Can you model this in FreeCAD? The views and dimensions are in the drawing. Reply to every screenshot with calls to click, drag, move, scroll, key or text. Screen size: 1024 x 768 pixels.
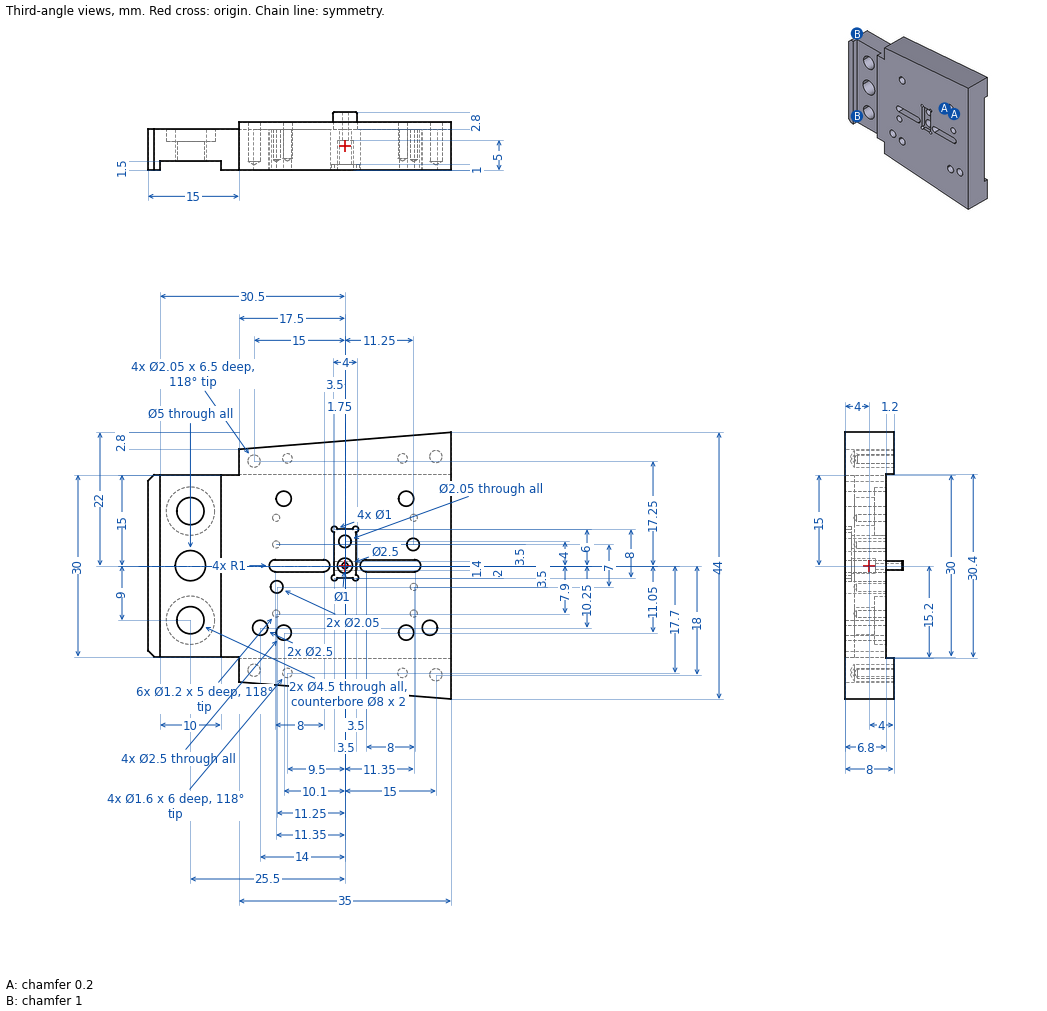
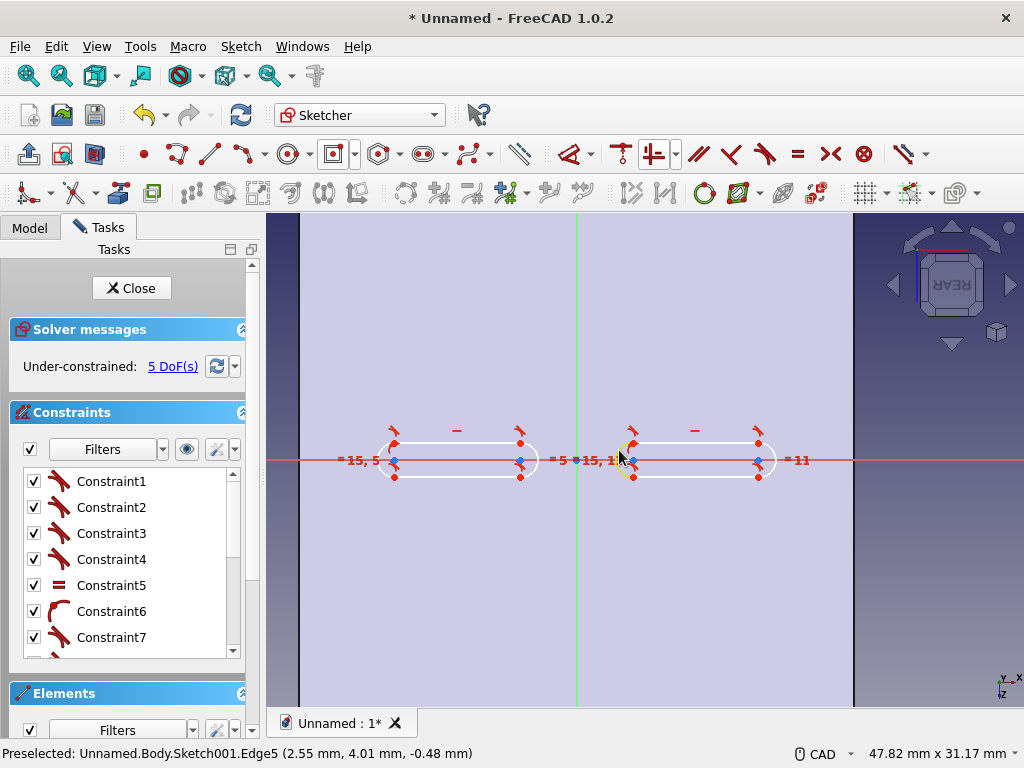
scroll(381, 450, up, 5)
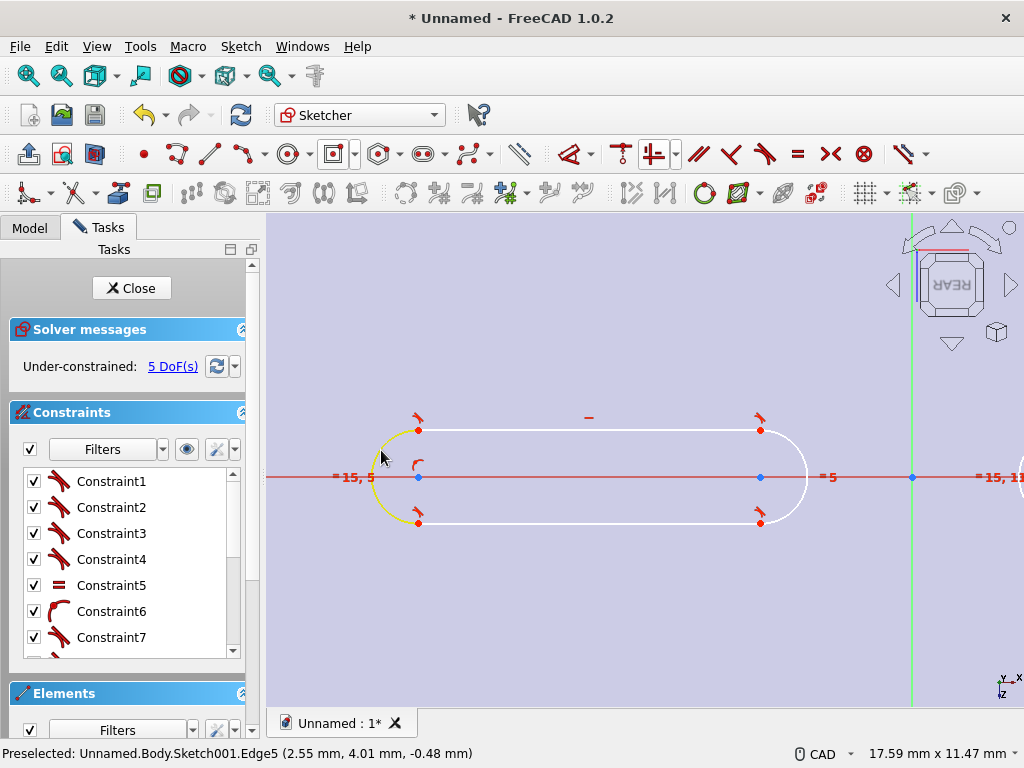
click(381, 450)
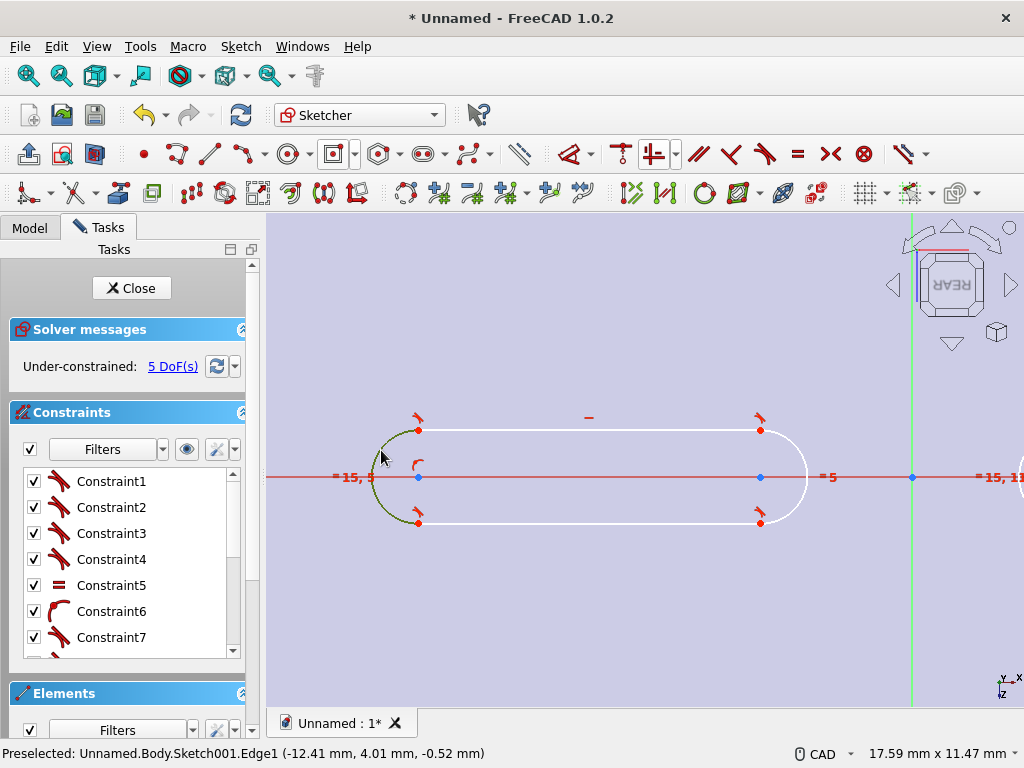
key(k)
key(r)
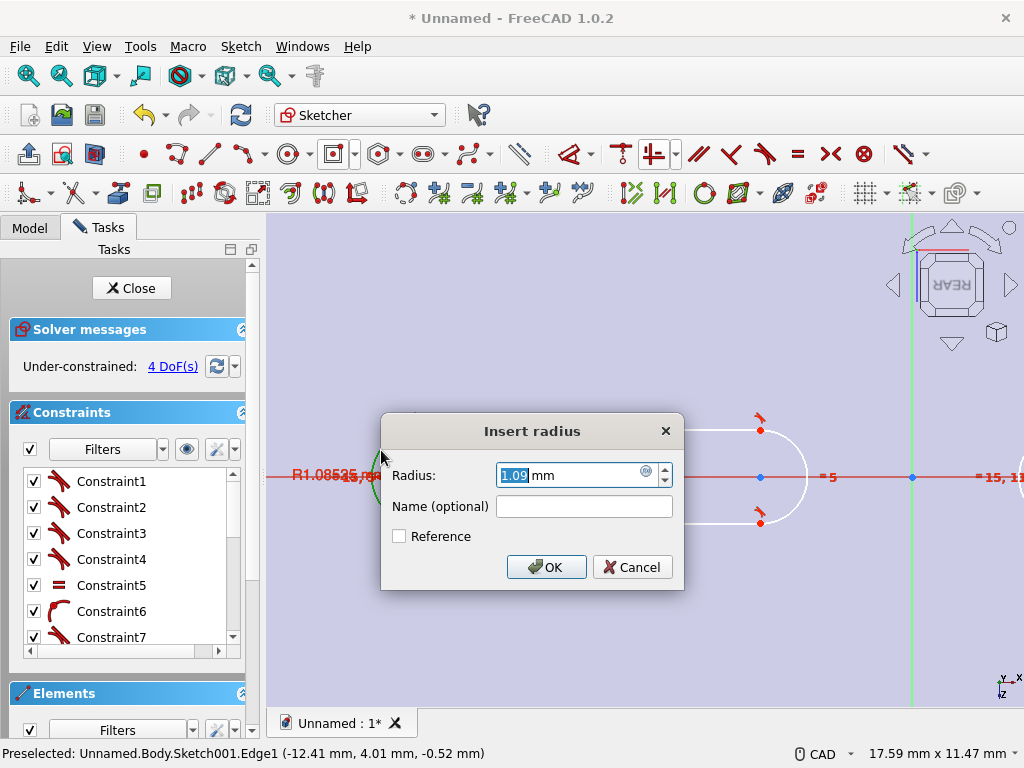
text(1)
key(Return)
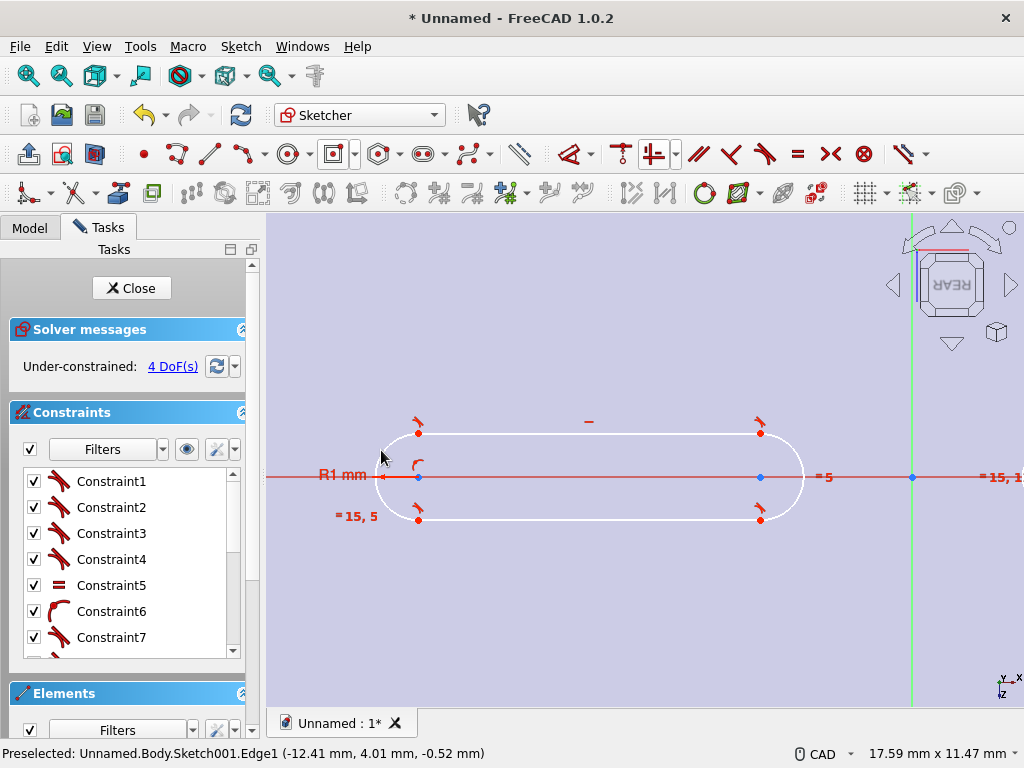
click(521, 434)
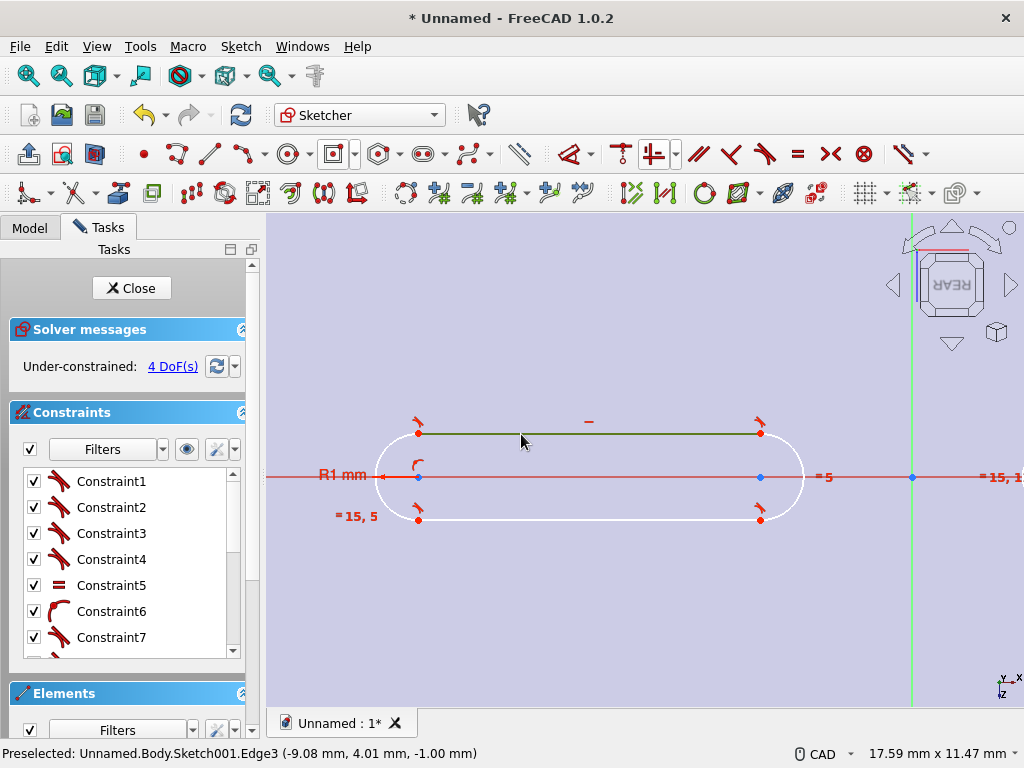
key(l)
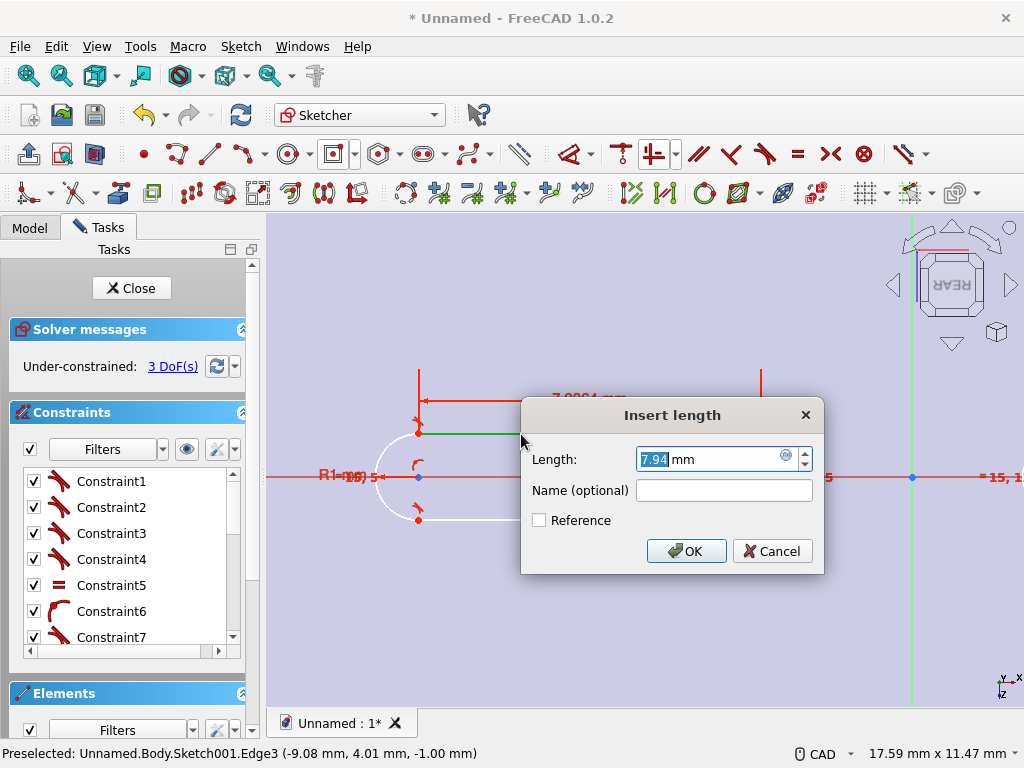
text(8)
key(Return)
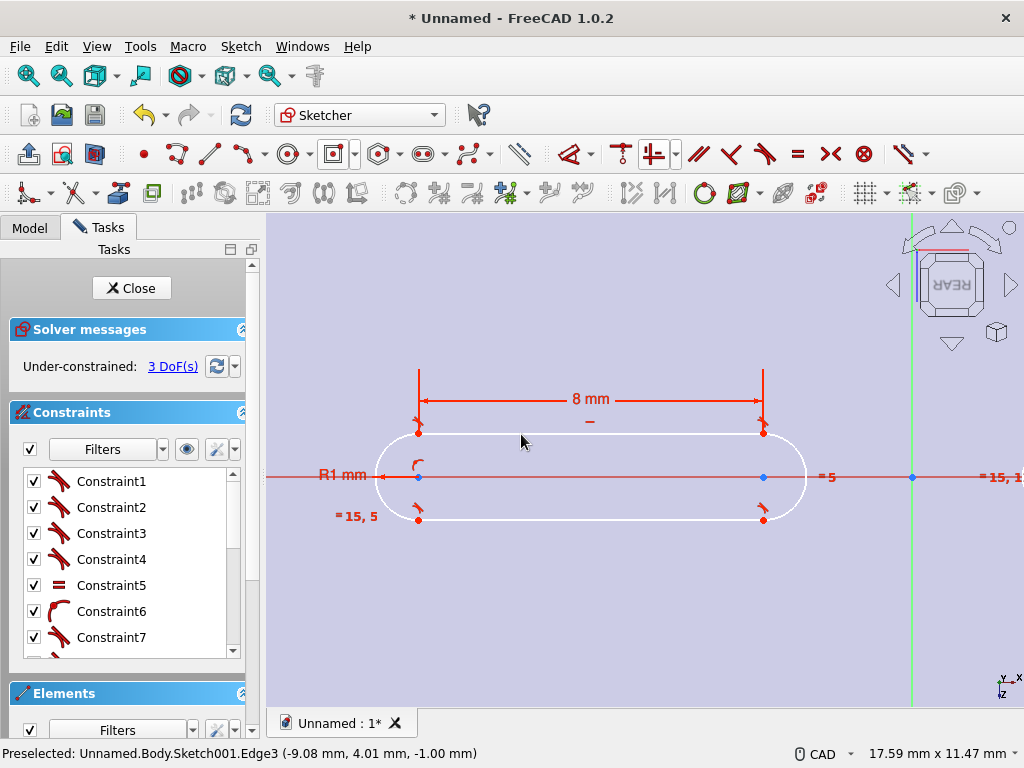
scroll(381, 450, down, 5)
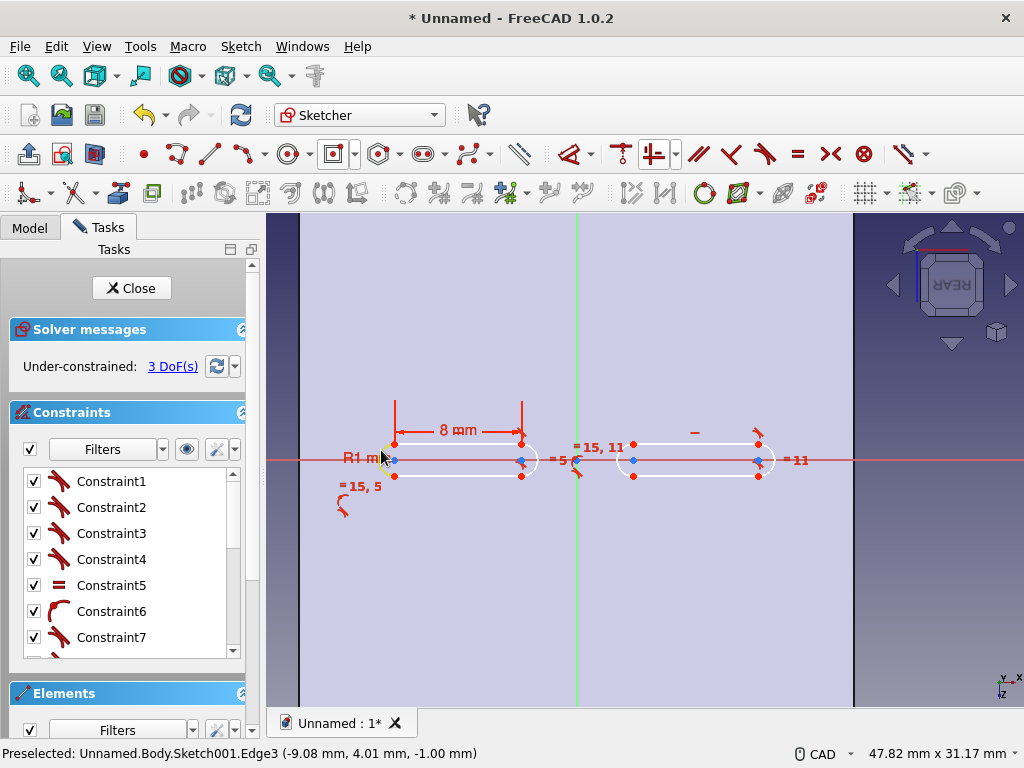
click(671, 444)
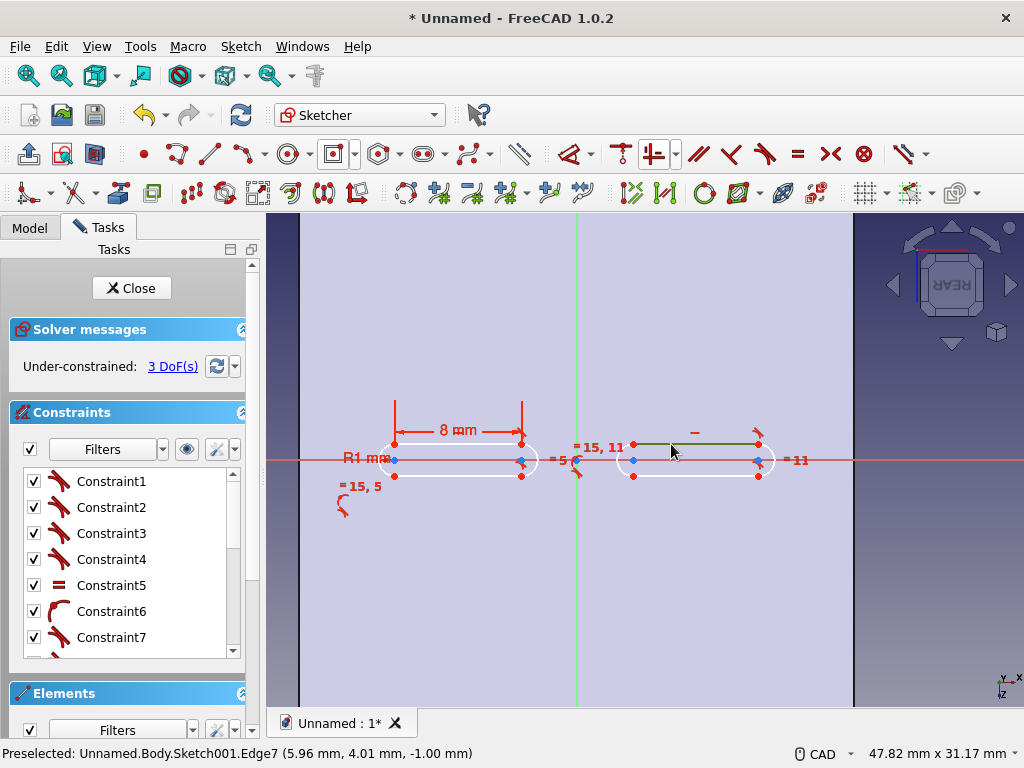
key(l)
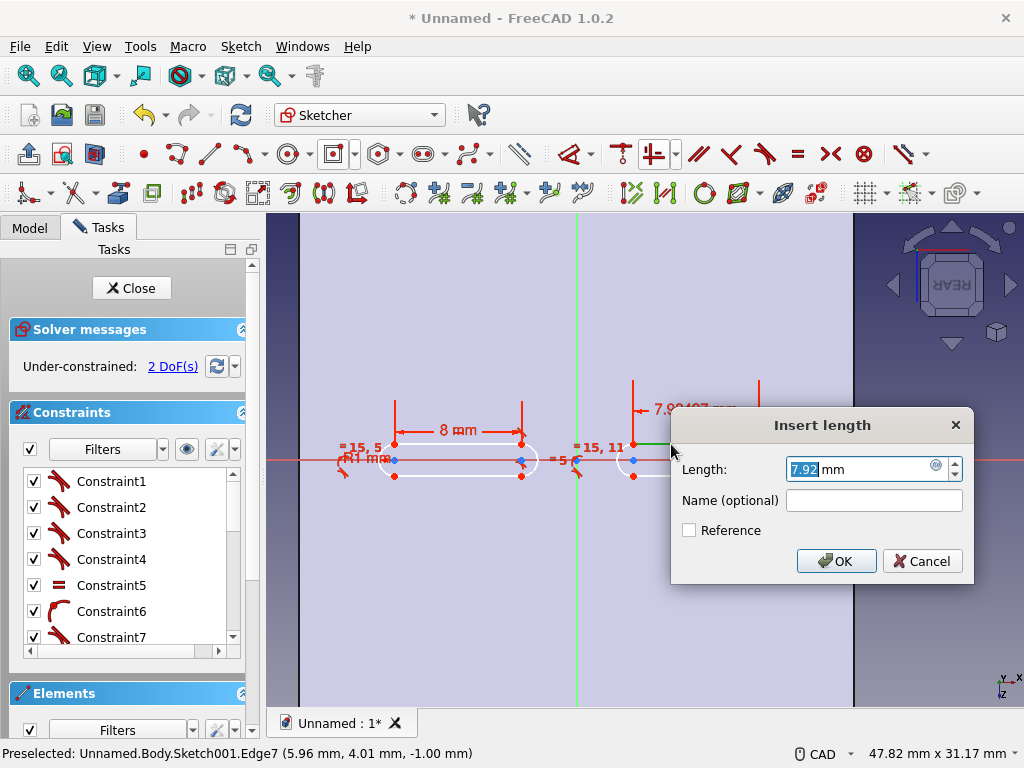
text(8)
key(Return)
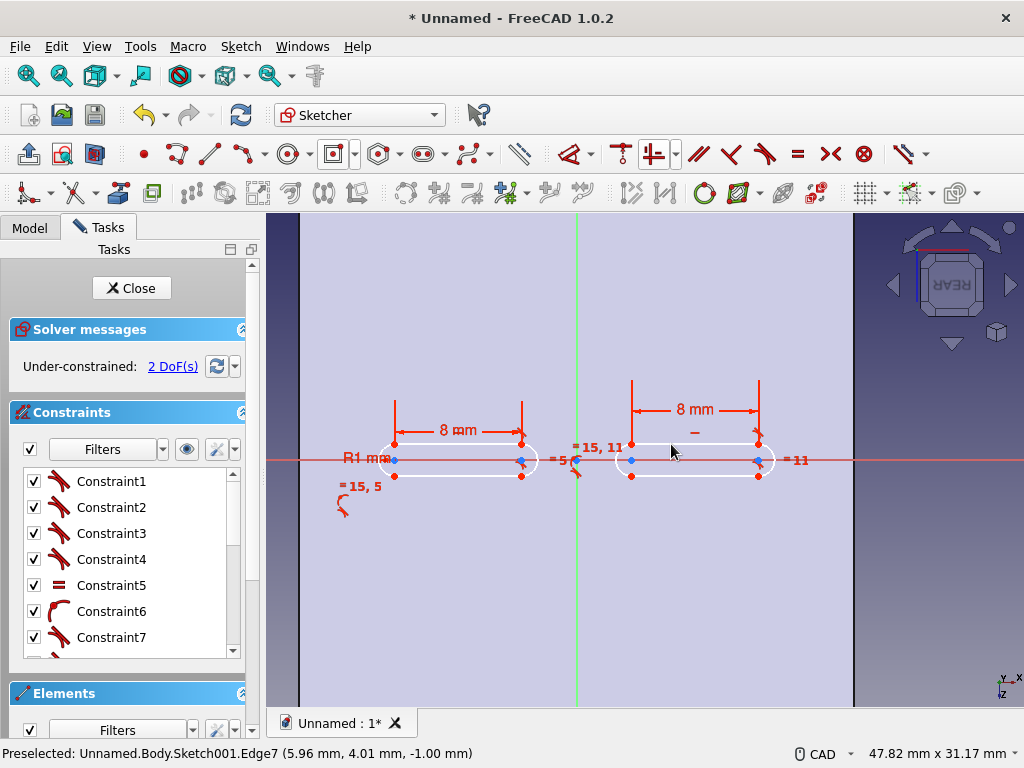
click(522, 476)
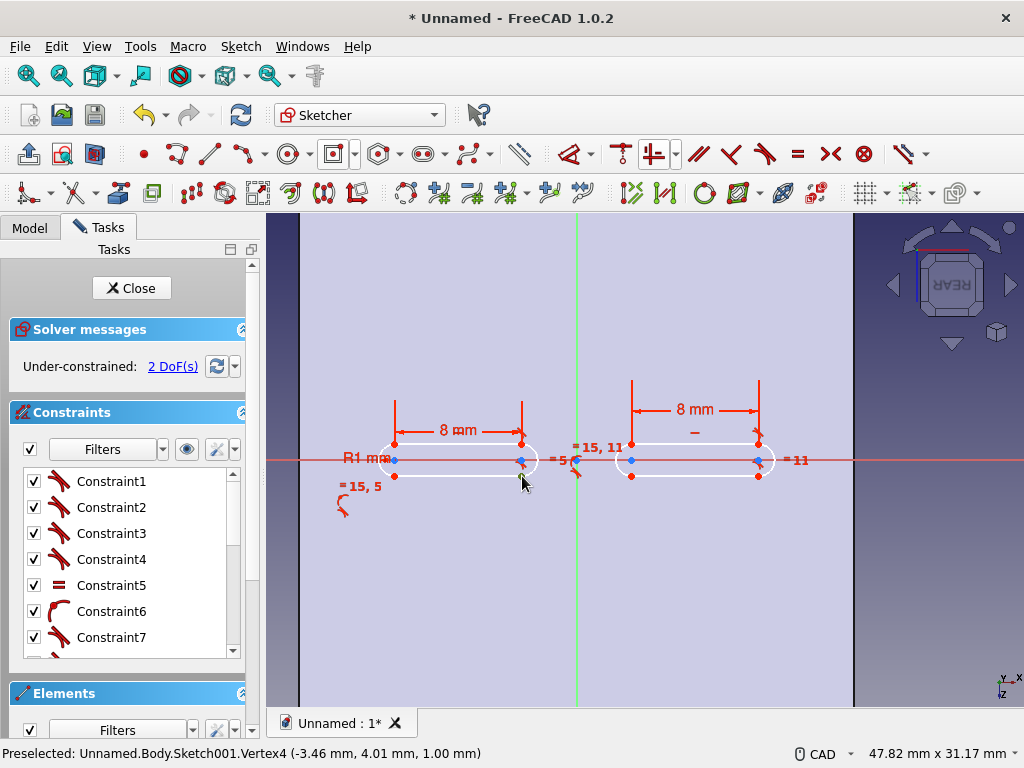
click(590, 154)